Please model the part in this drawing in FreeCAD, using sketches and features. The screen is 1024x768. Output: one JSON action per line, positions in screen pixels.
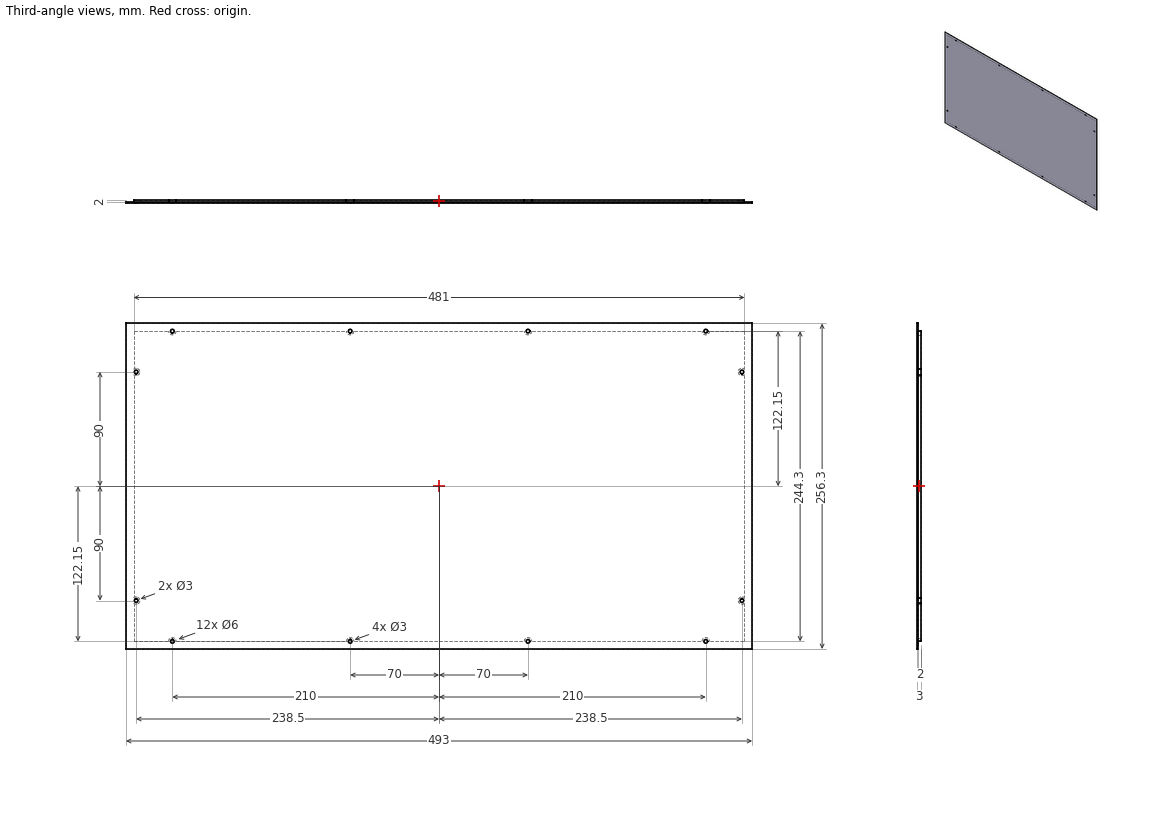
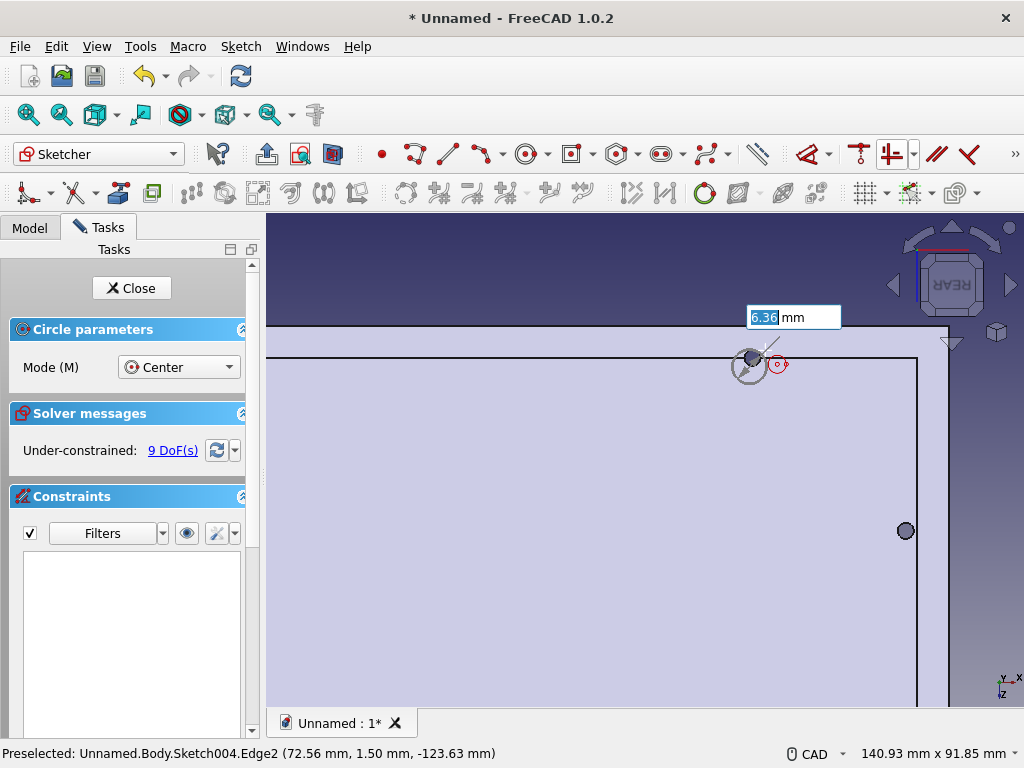
{"action": "left_click", "coordinate": [764, 347]}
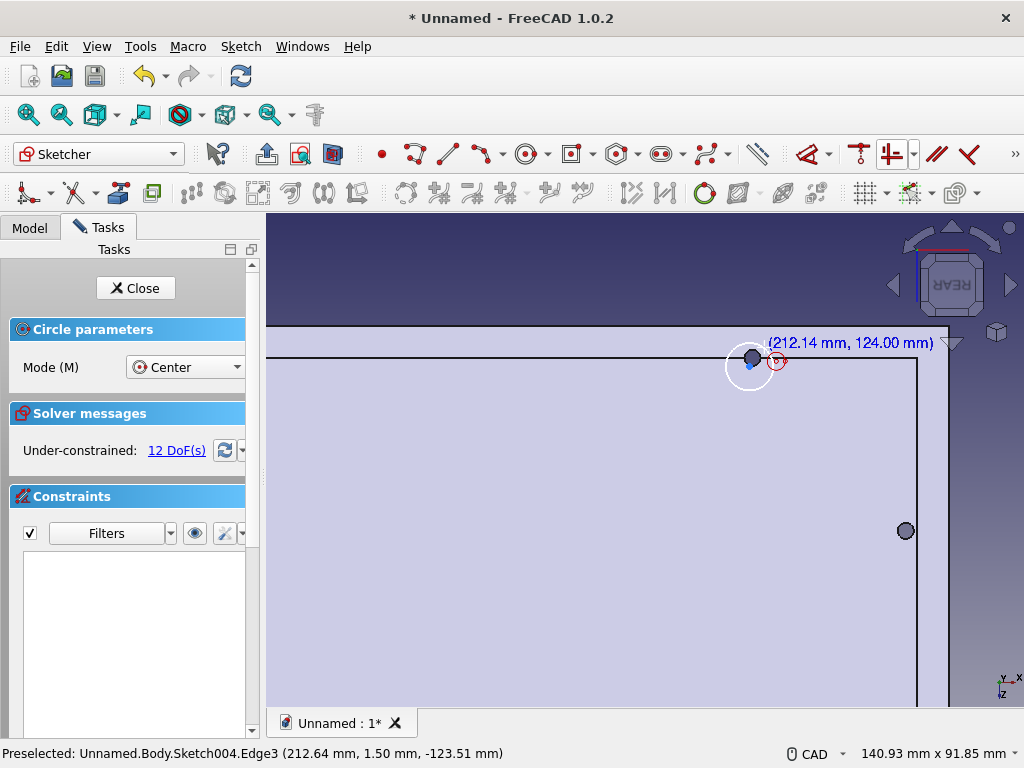
{"action": "scroll", "coordinate": [765, 350], "scroll_direction": "down", "scroll_amount": 9}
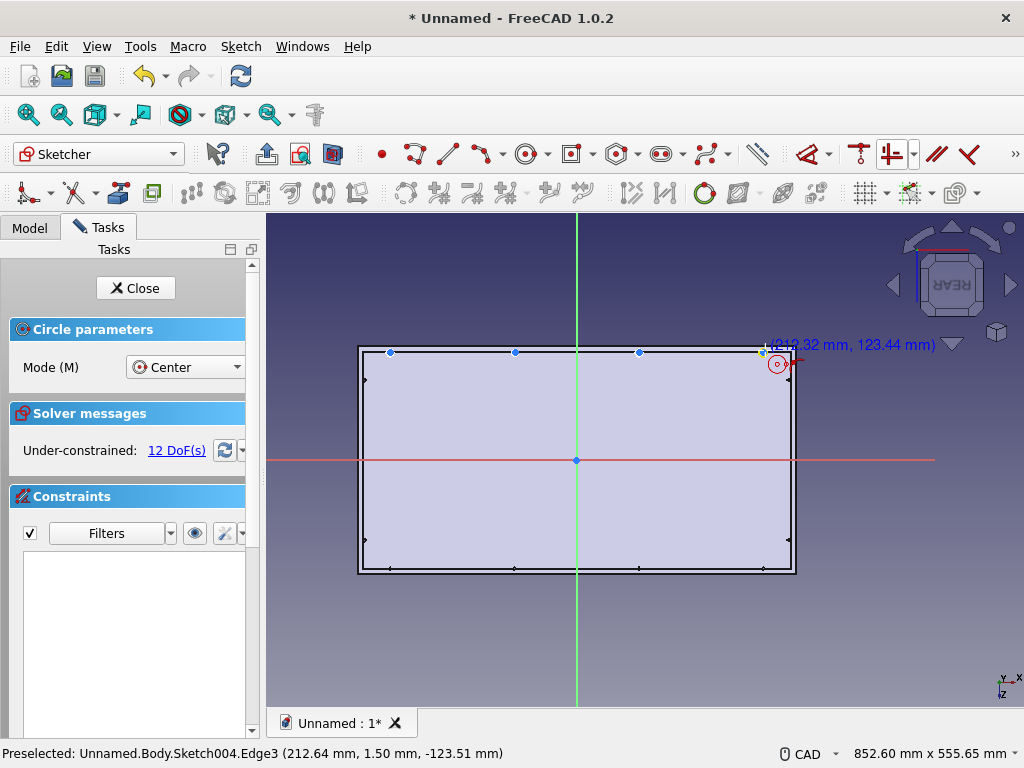
{"action": "scroll", "coordinate": [789, 380], "scroll_direction": "up", "scroll_amount": 11}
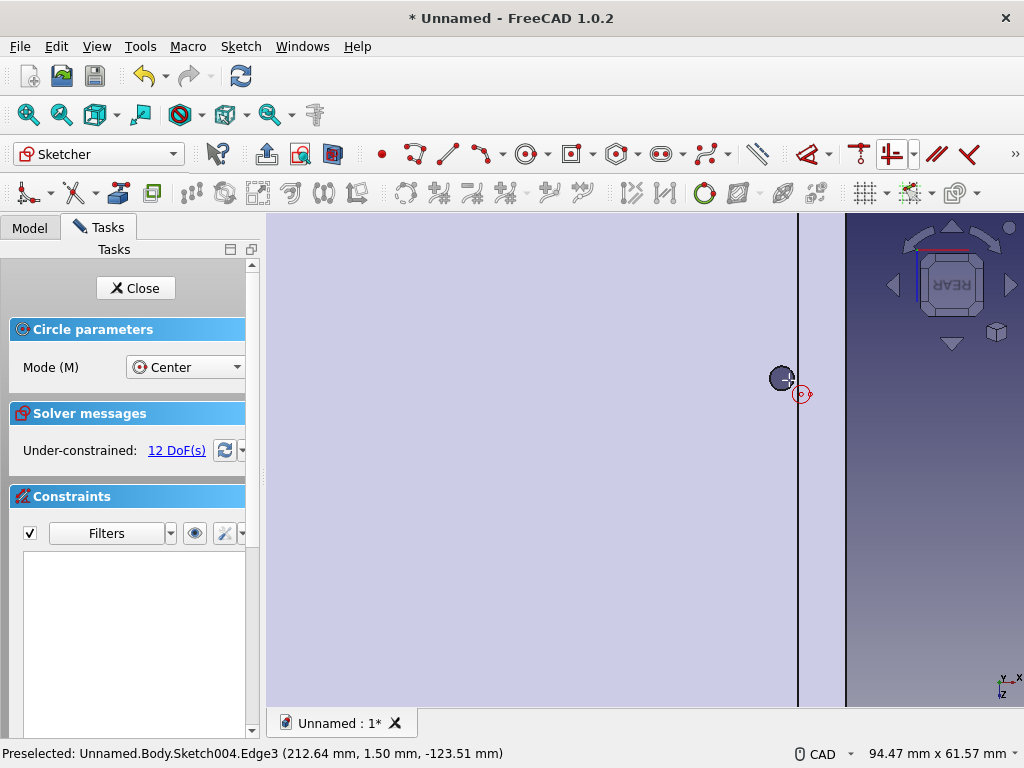
{"action": "scroll", "coordinate": [789, 380], "scroll_direction": "down", "scroll_amount": 11}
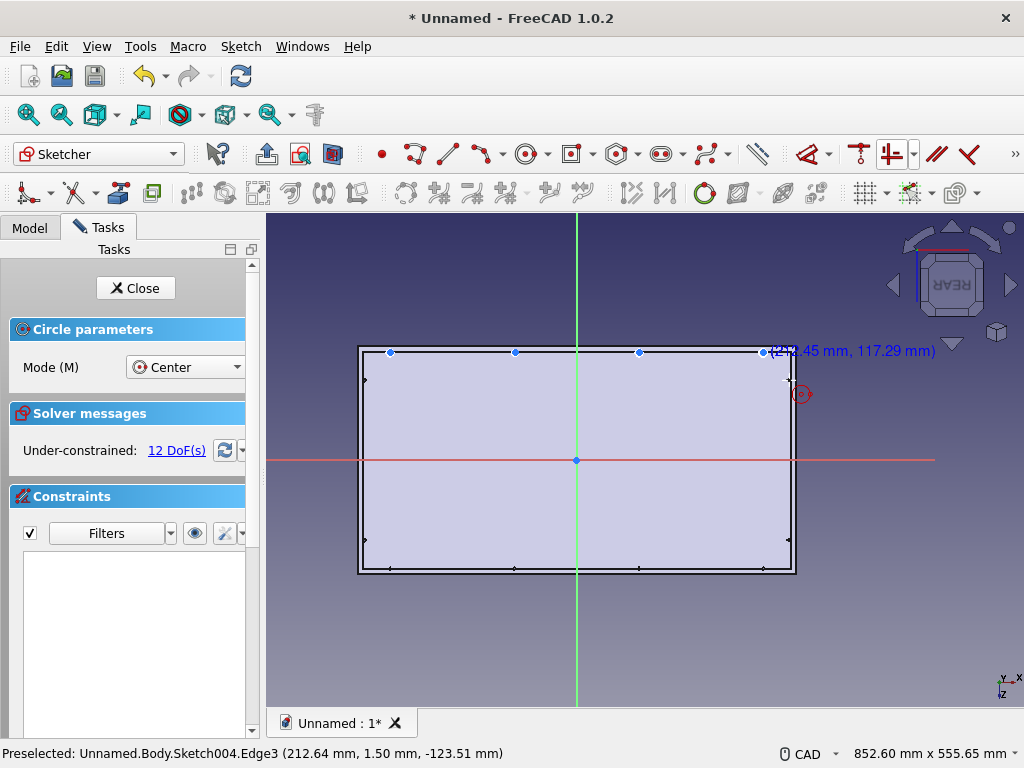
{"action": "left_click", "coordinate": [789, 380]}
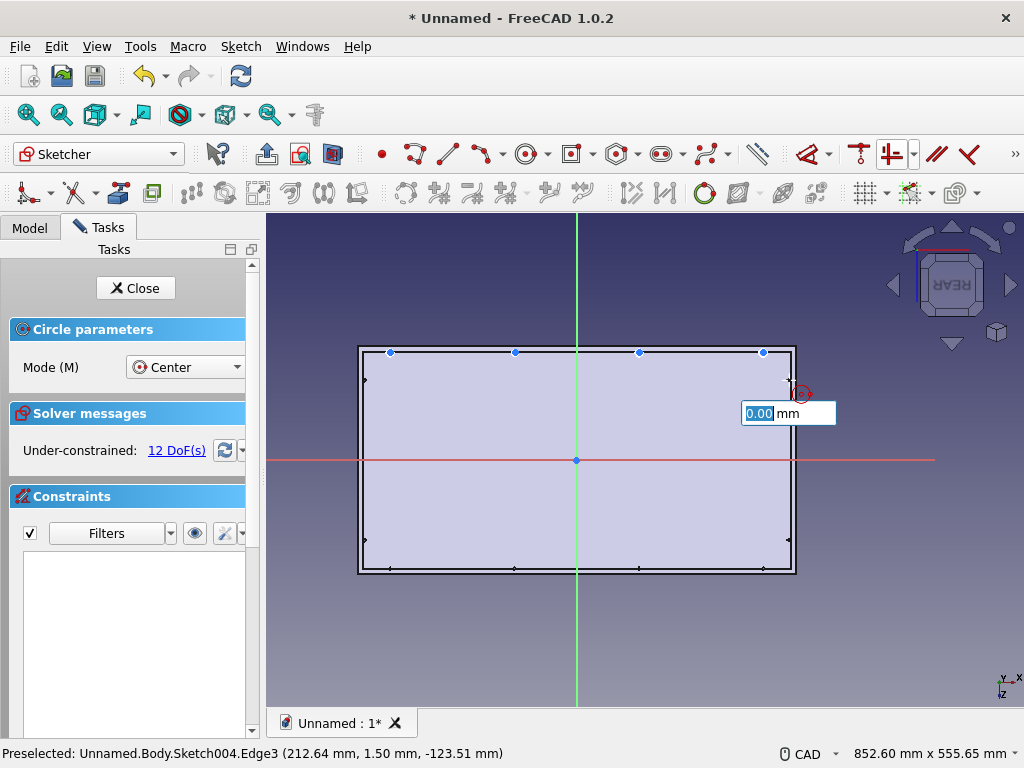
{"action": "scroll", "coordinate": [791, 378], "scroll_direction": "up", "scroll_amount": 9}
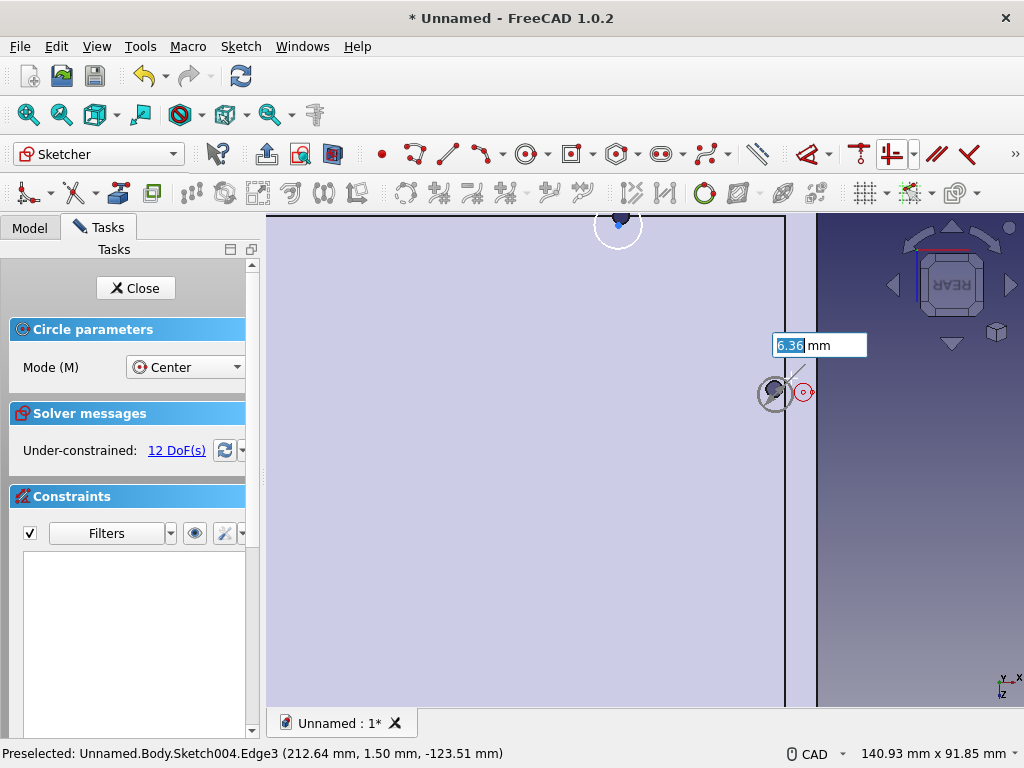
{"action": "left_click", "coordinate": [786, 378]}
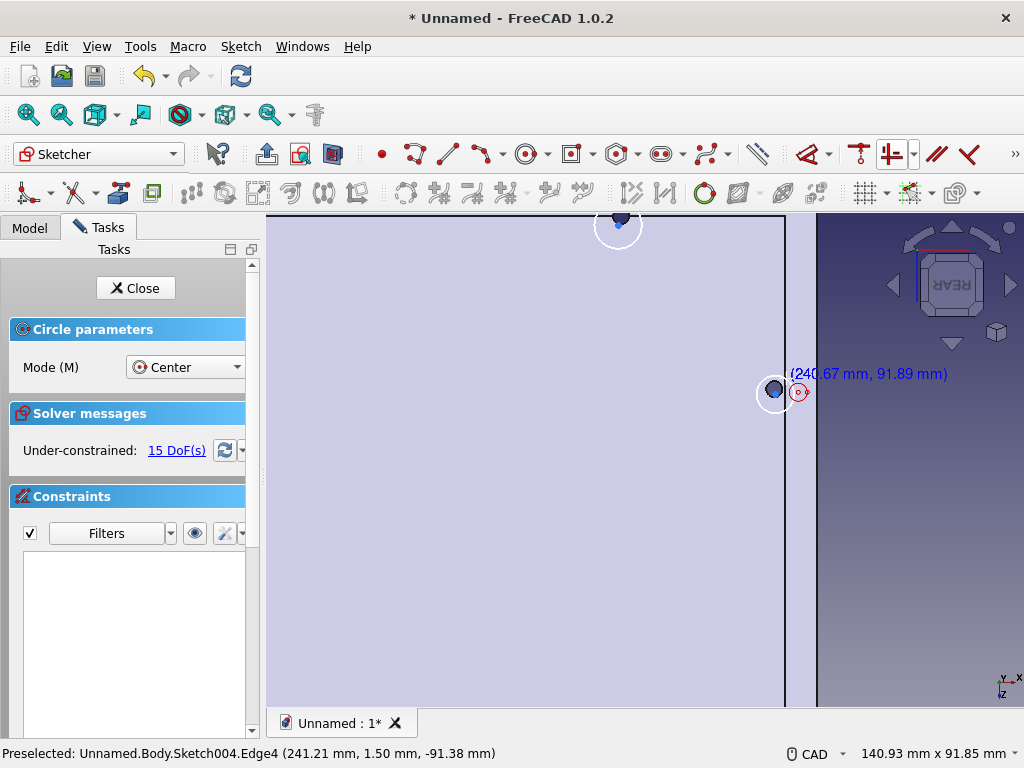
{"action": "scroll", "coordinate": [791, 378], "scroll_direction": "down", "scroll_amount": 9}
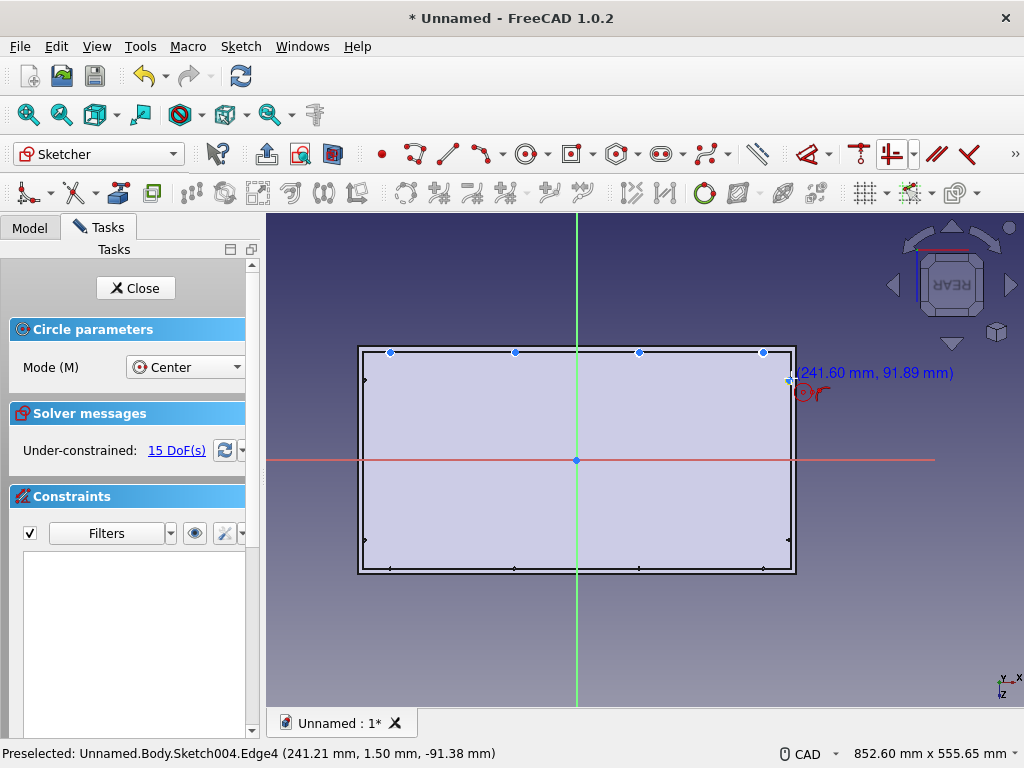
{"action": "scroll", "coordinate": [789, 540], "scroll_direction": "up", "scroll_amount": 11}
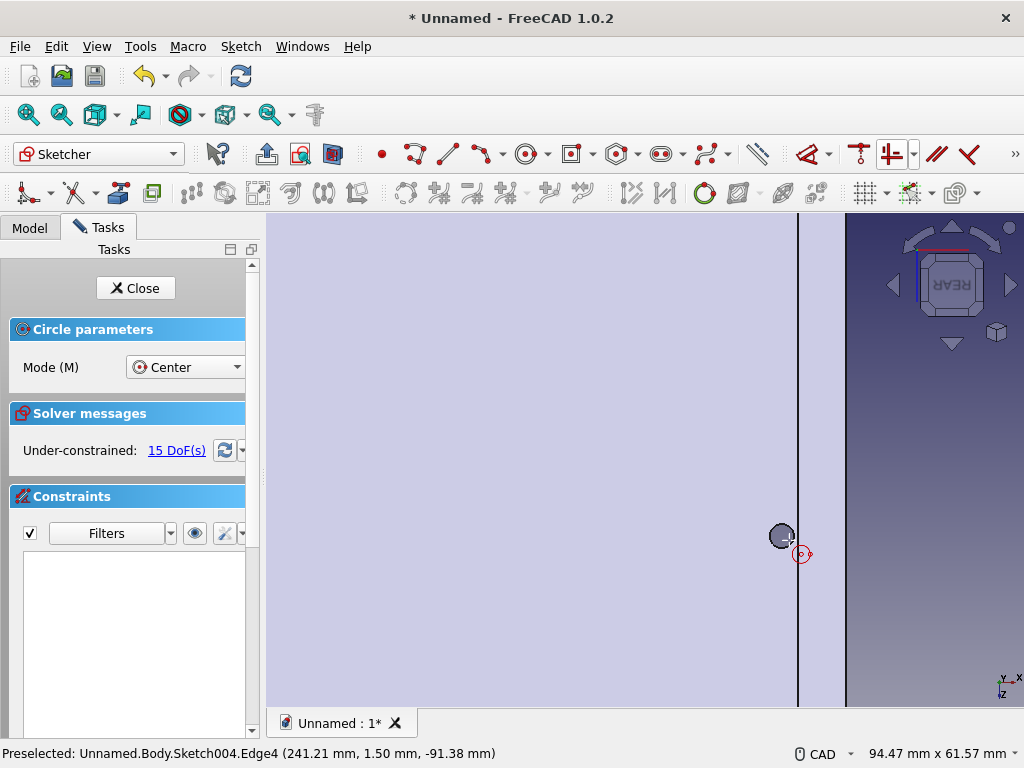
{"action": "scroll", "coordinate": [789, 541], "scroll_direction": "down", "scroll_amount": 11}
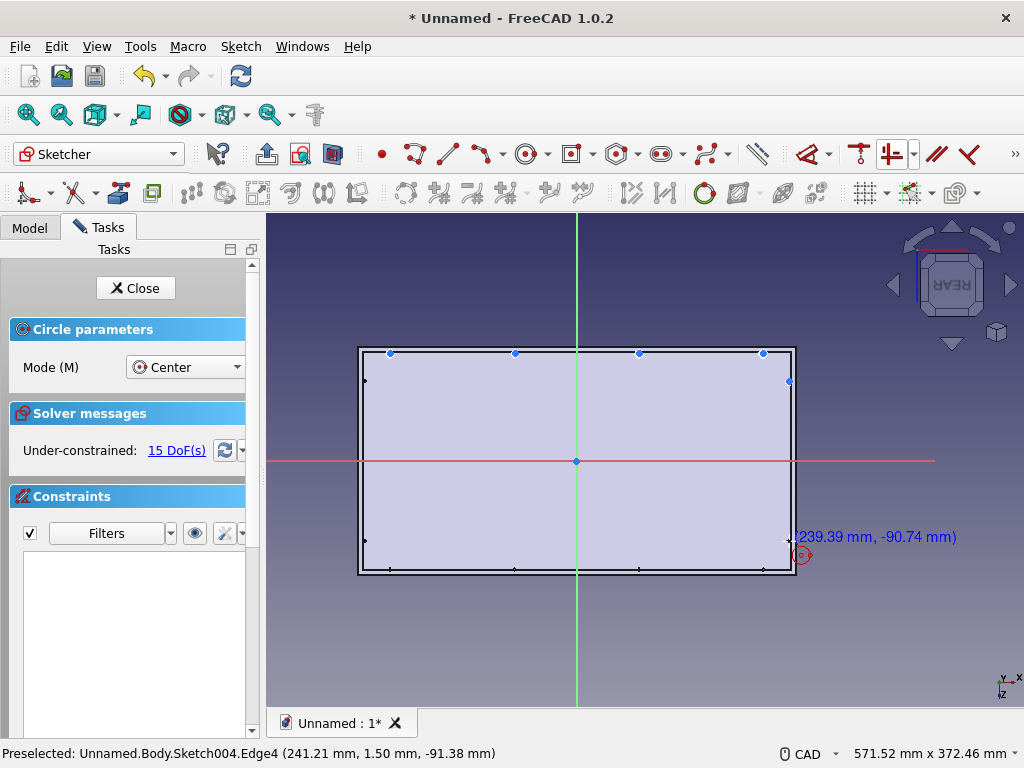
{"action": "left_click", "coordinate": [789, 541]}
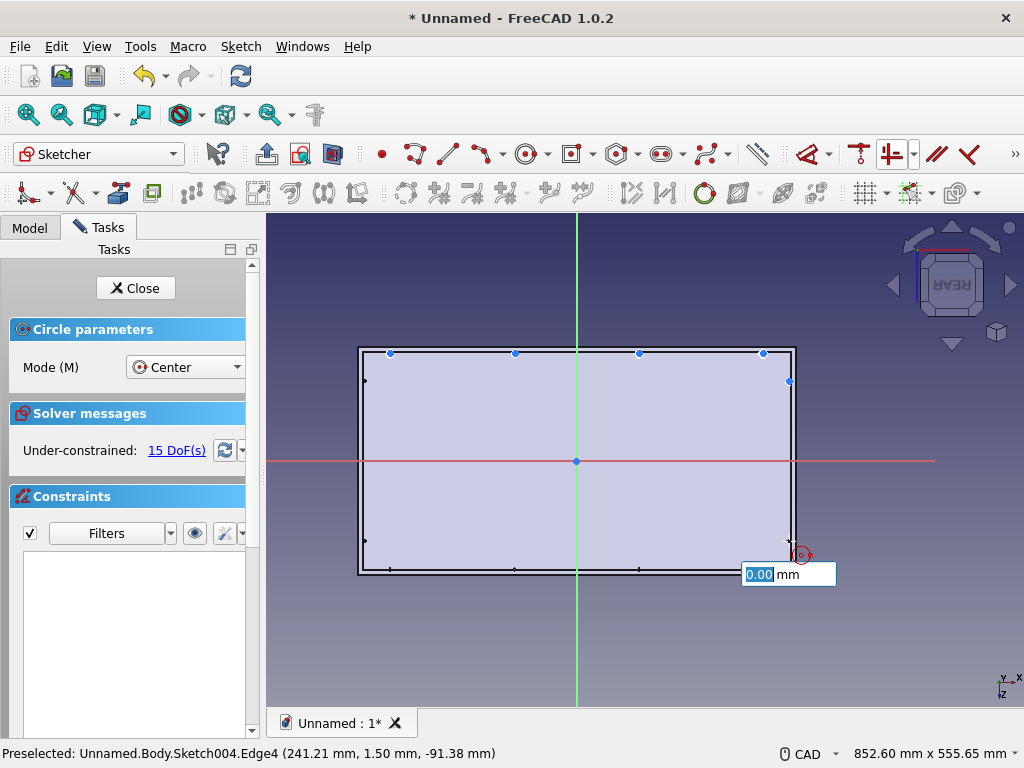
{"action": "scroll", "coordinate": [791, 539], "scroll_direction": "up", "scroll_amount": 9}